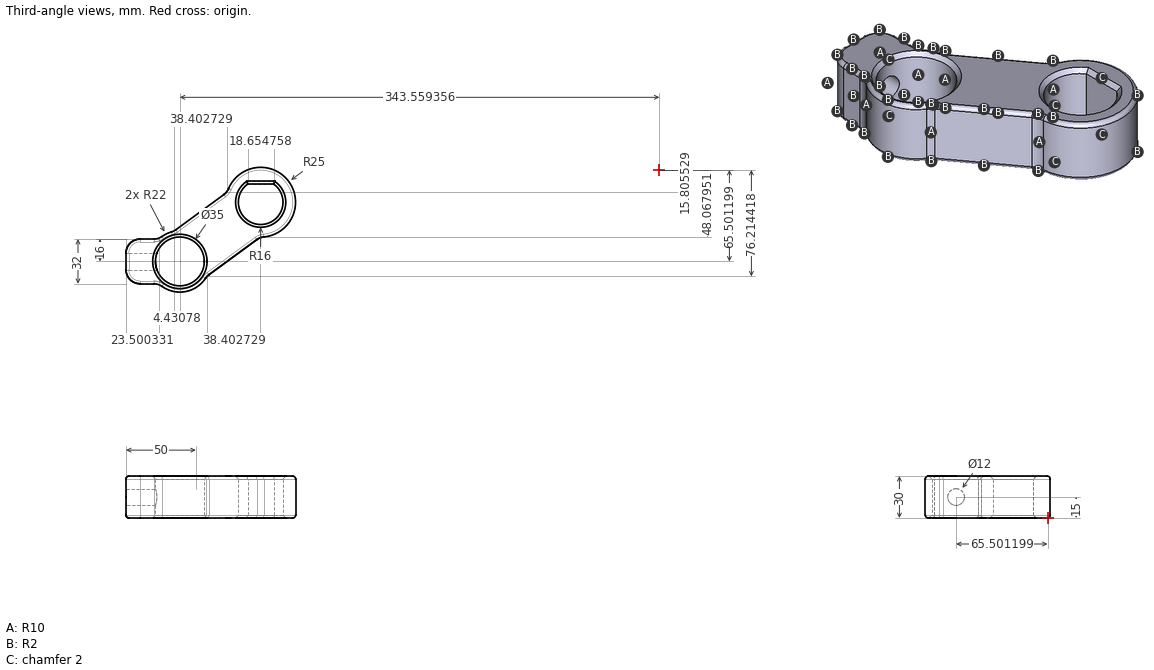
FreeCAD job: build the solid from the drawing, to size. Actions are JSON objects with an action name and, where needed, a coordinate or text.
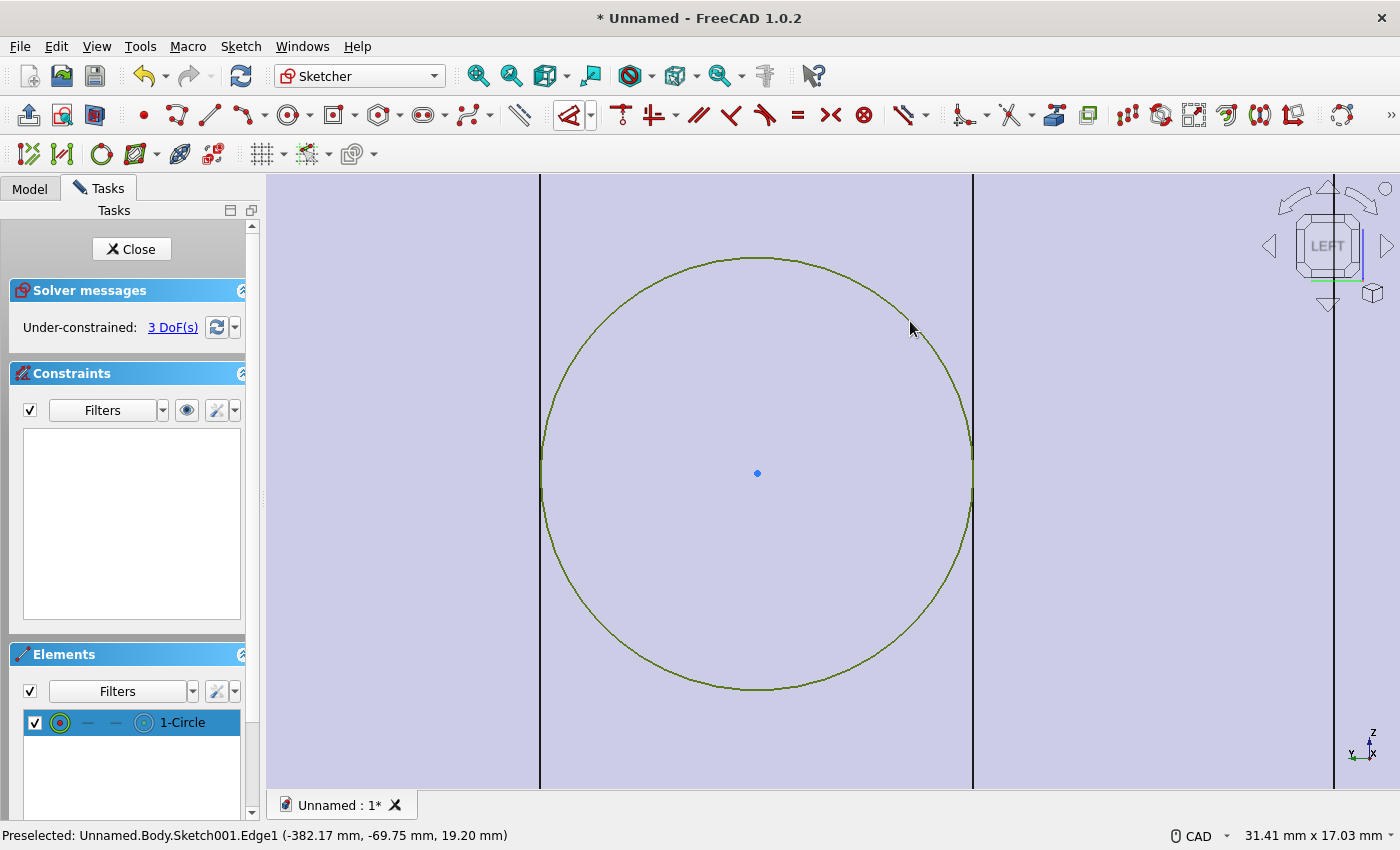
{"action": "left_click", "coordinate": [590, 116]}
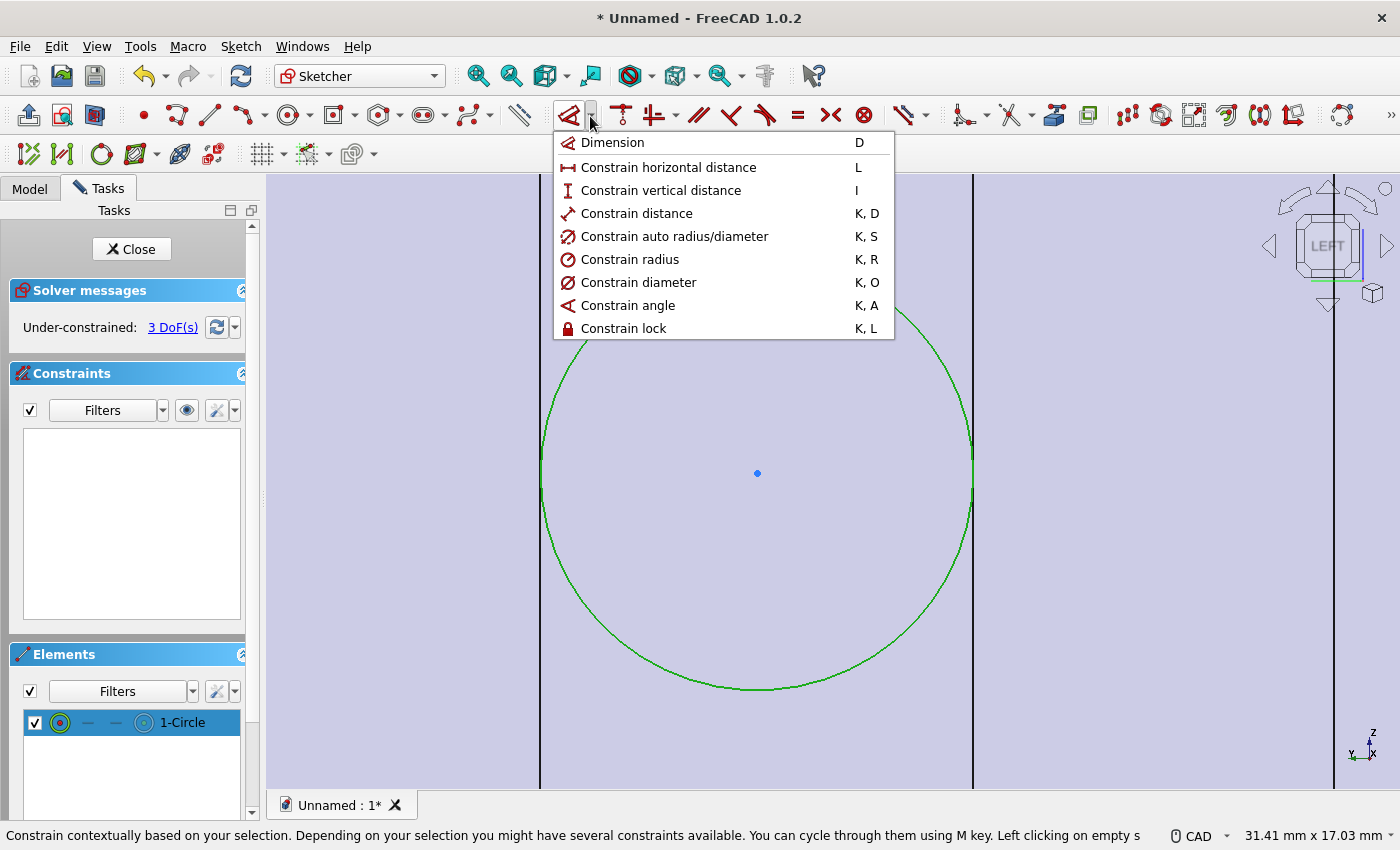
{"action": "left_click", "coordinate": [724, 282]}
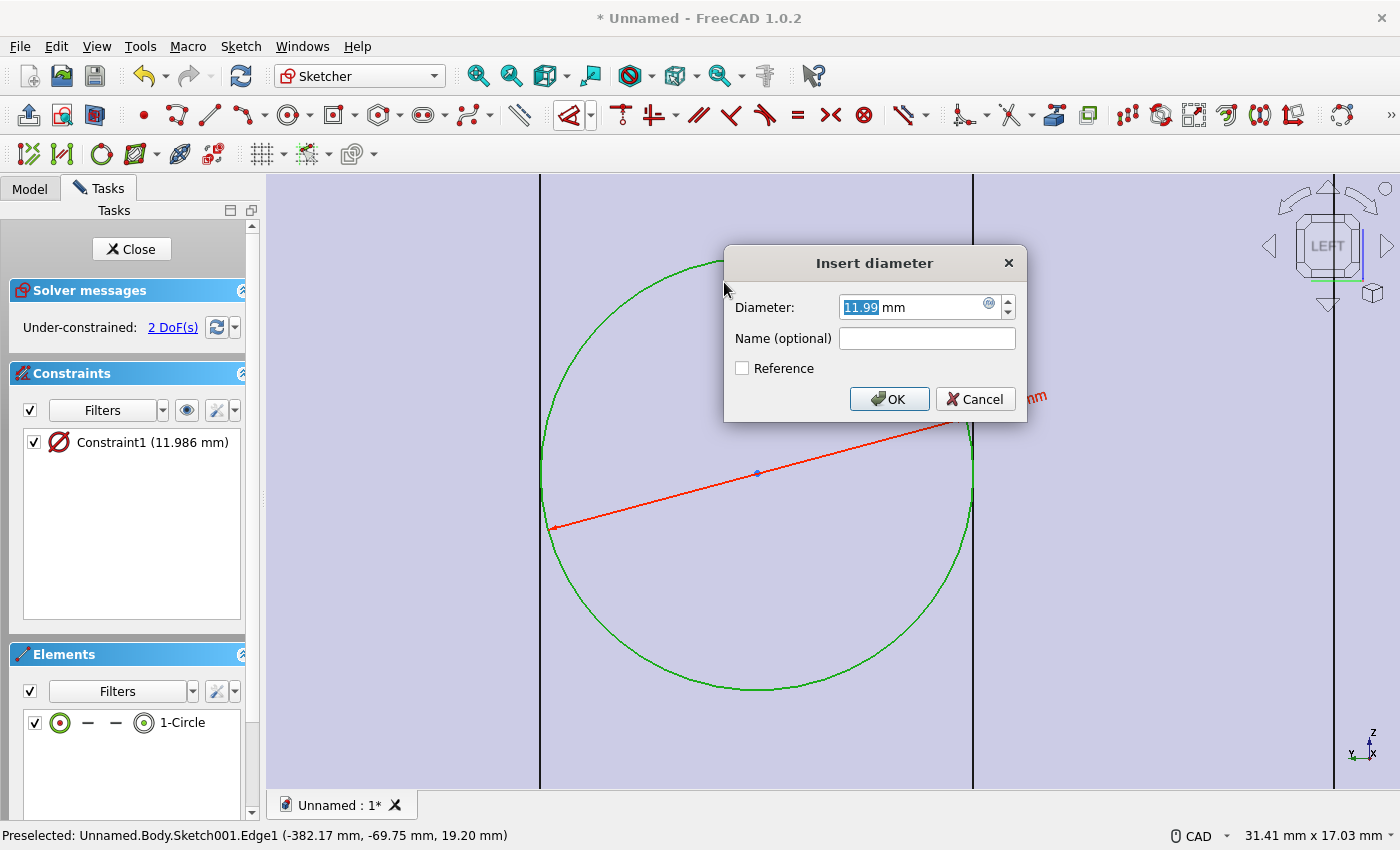
{"action": "type", "text": "12"}
{"action": "key", "text": "Return"}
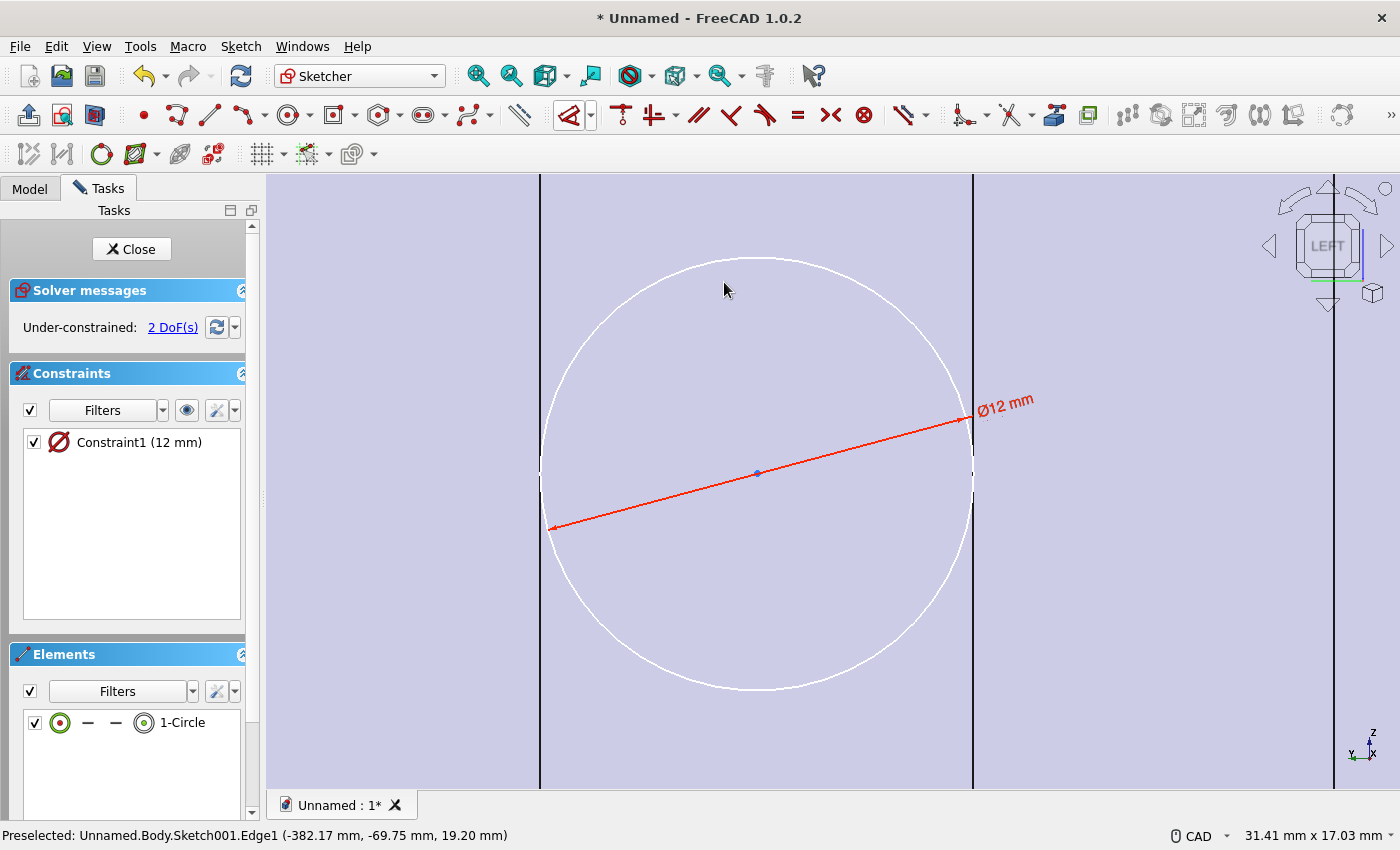
{"action": "left_click", "coordinate": [757, 474]}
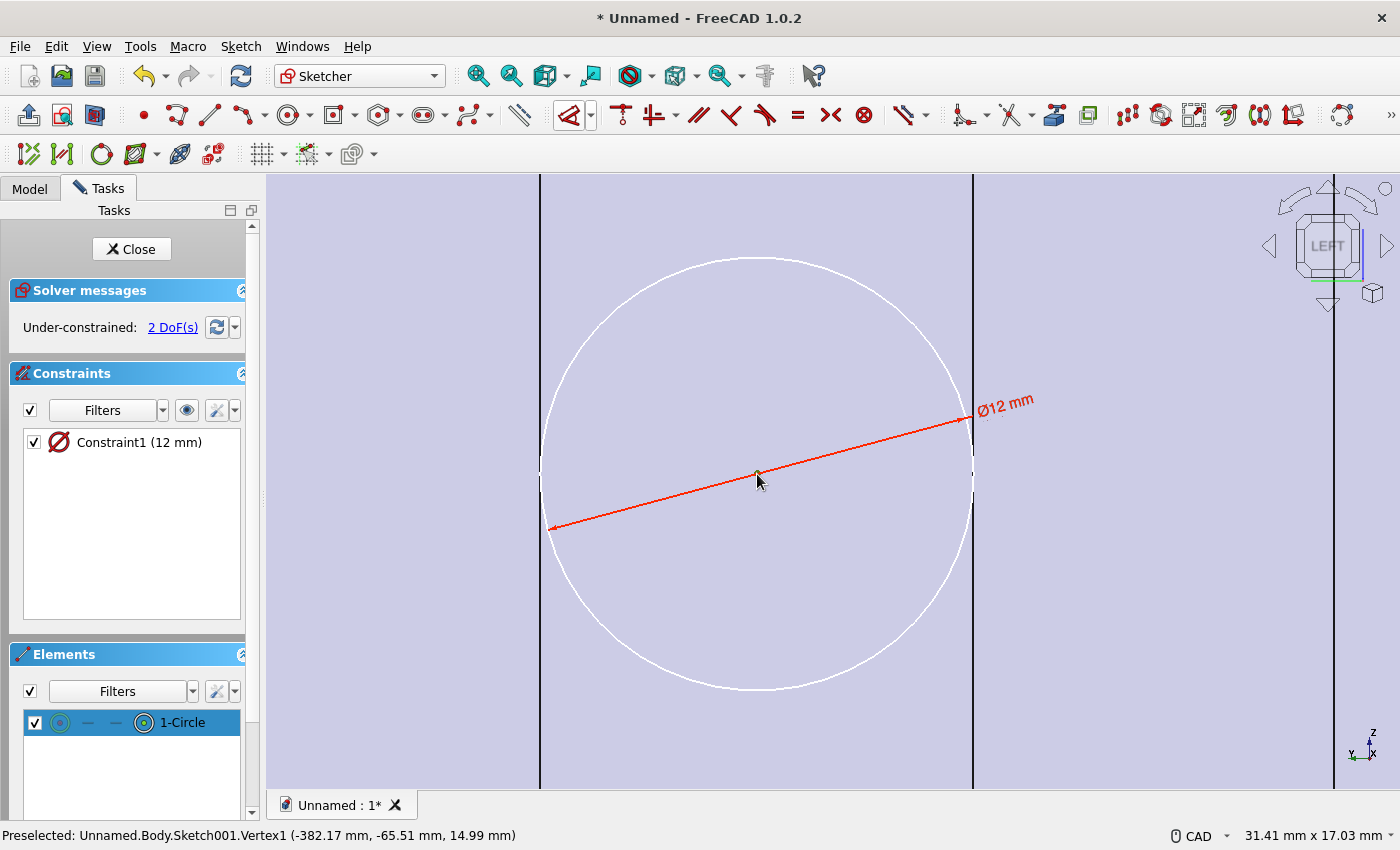
{"action": "key", "text": "i"}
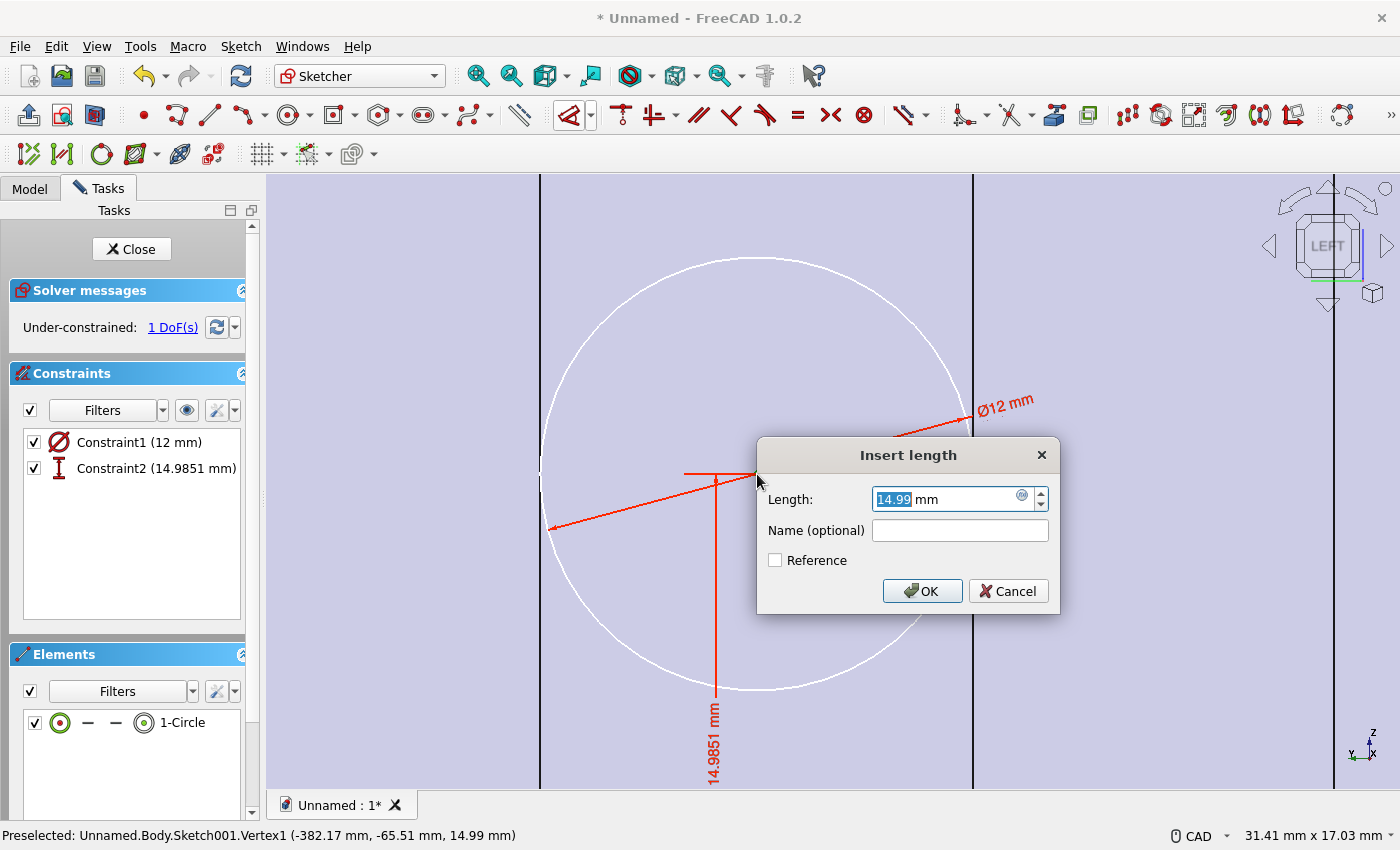
{"action": "type", "text": "15"}
{"action": "key", "text": "Return"}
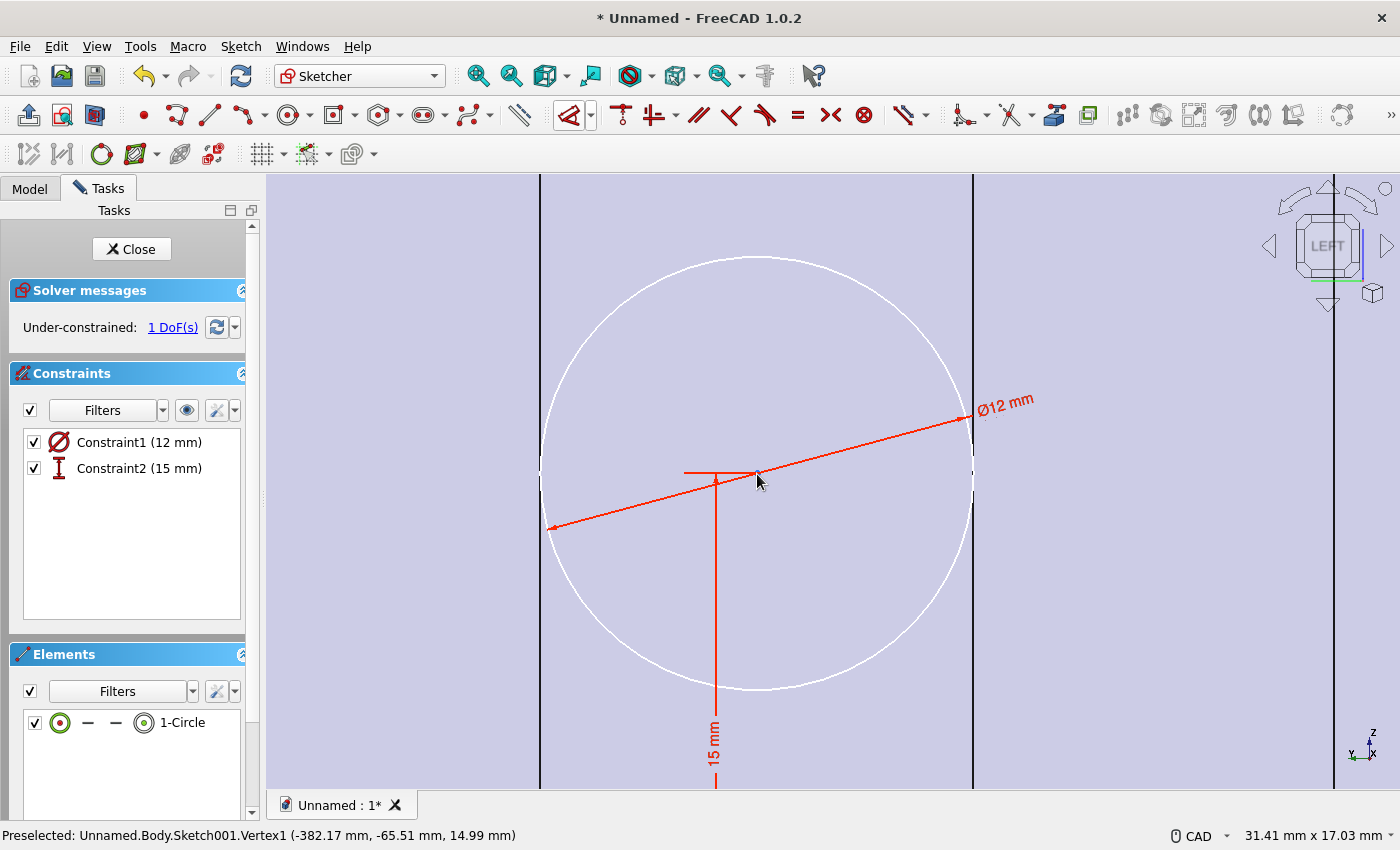
{"action": "left_click", "coordinate": [757, 473]}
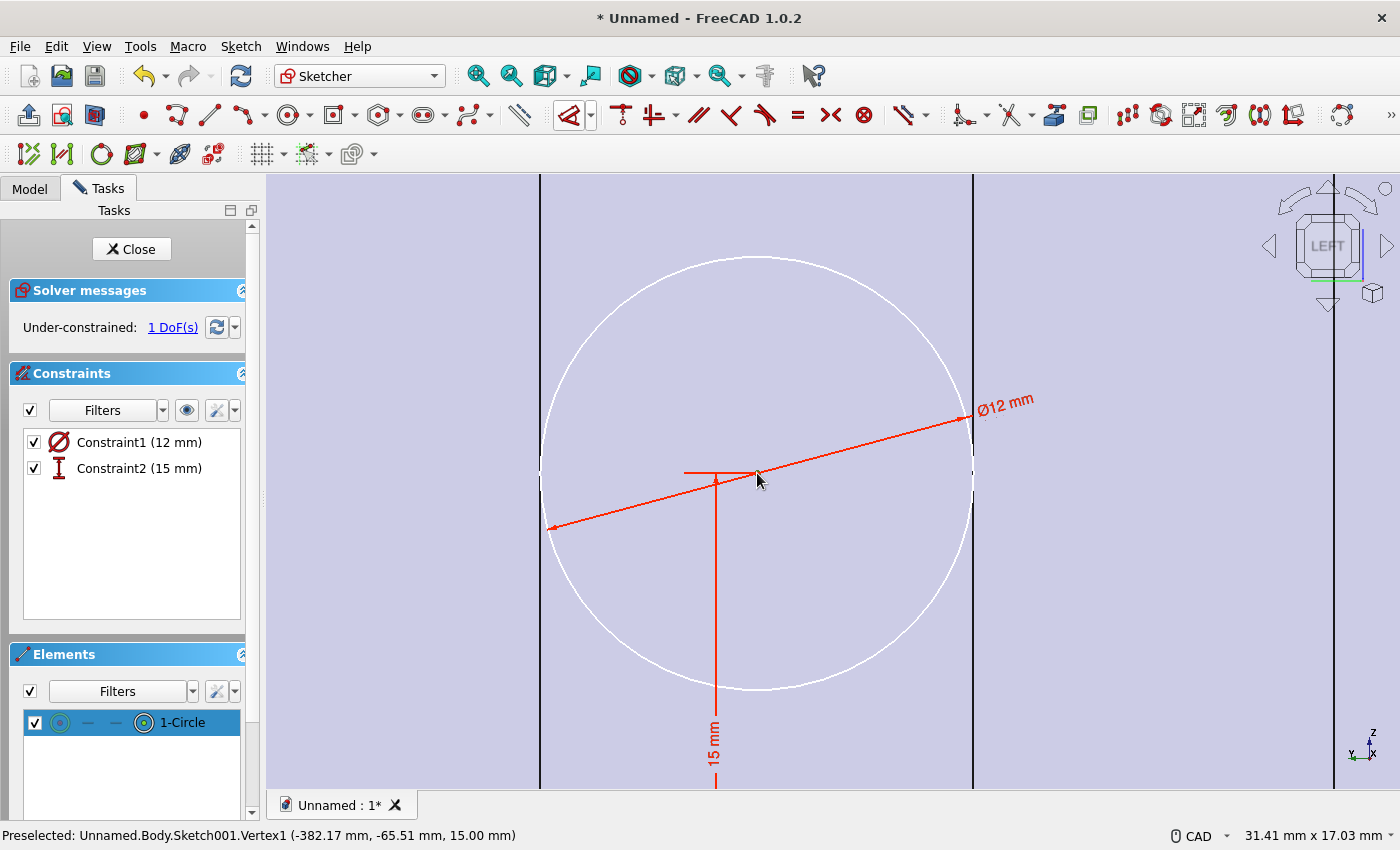
{"action": "left_click", "coordinate": [590, 116]}